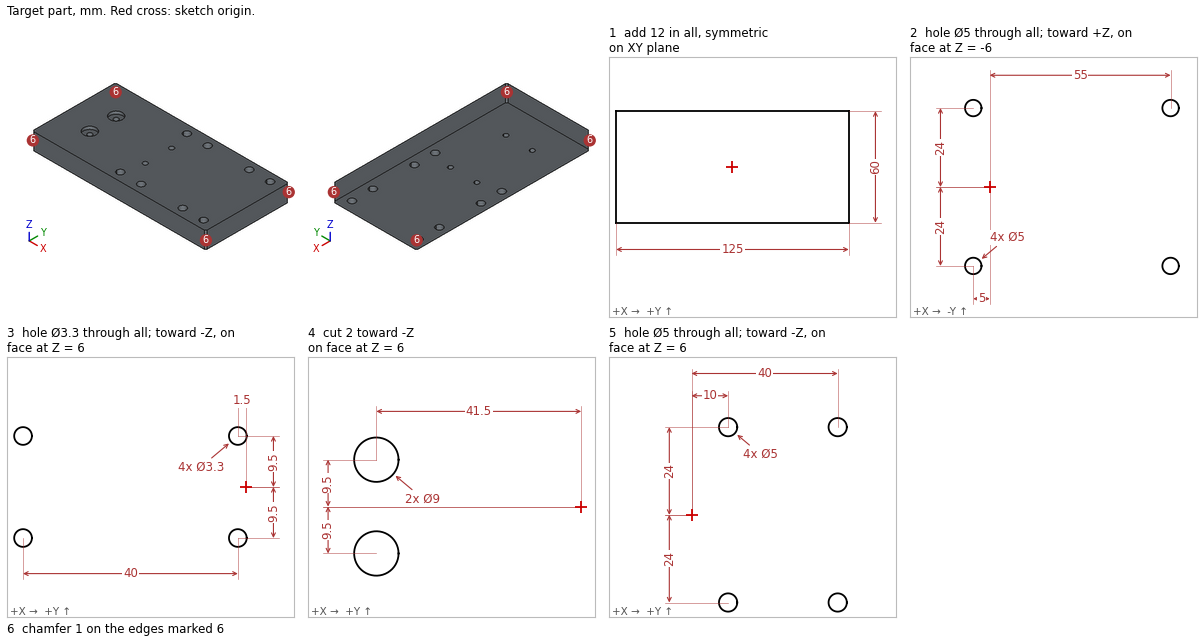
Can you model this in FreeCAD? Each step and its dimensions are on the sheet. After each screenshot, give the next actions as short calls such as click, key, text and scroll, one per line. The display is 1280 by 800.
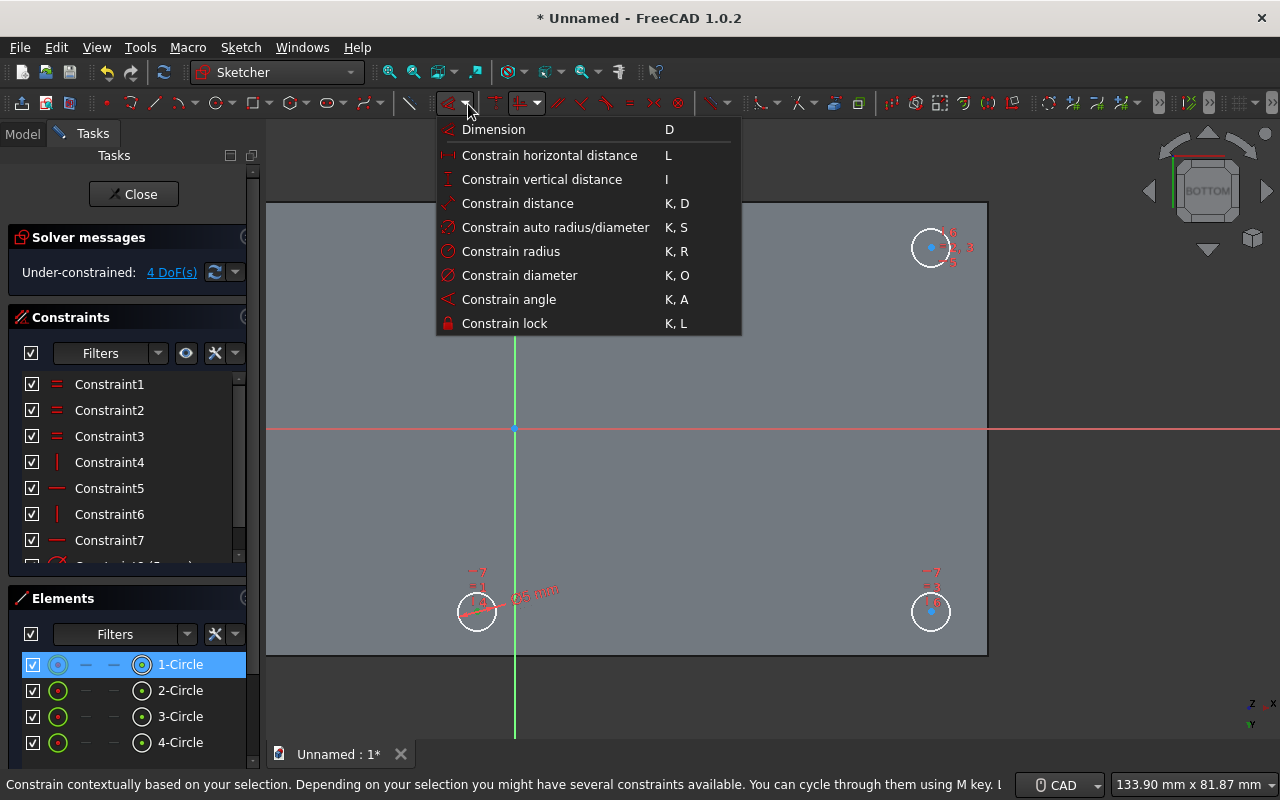
click(589, 155)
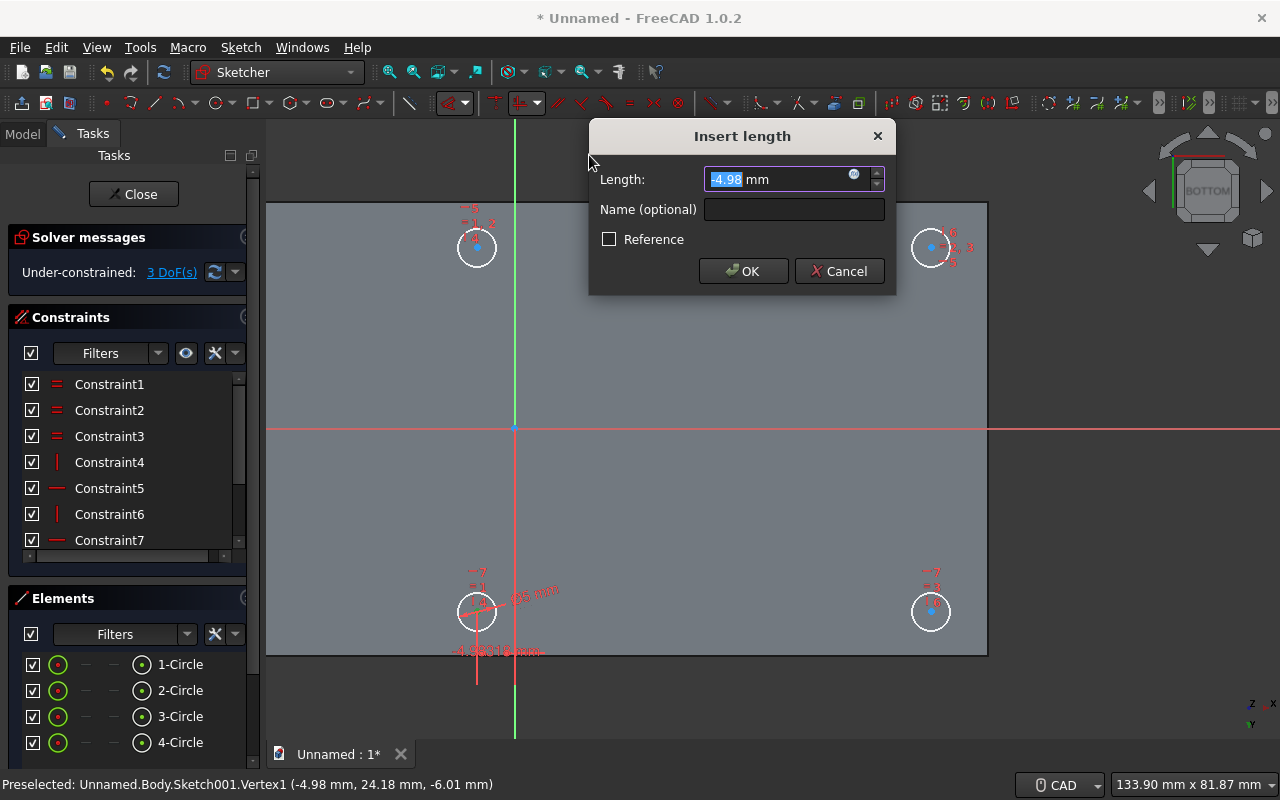
text(-5)
key(Return)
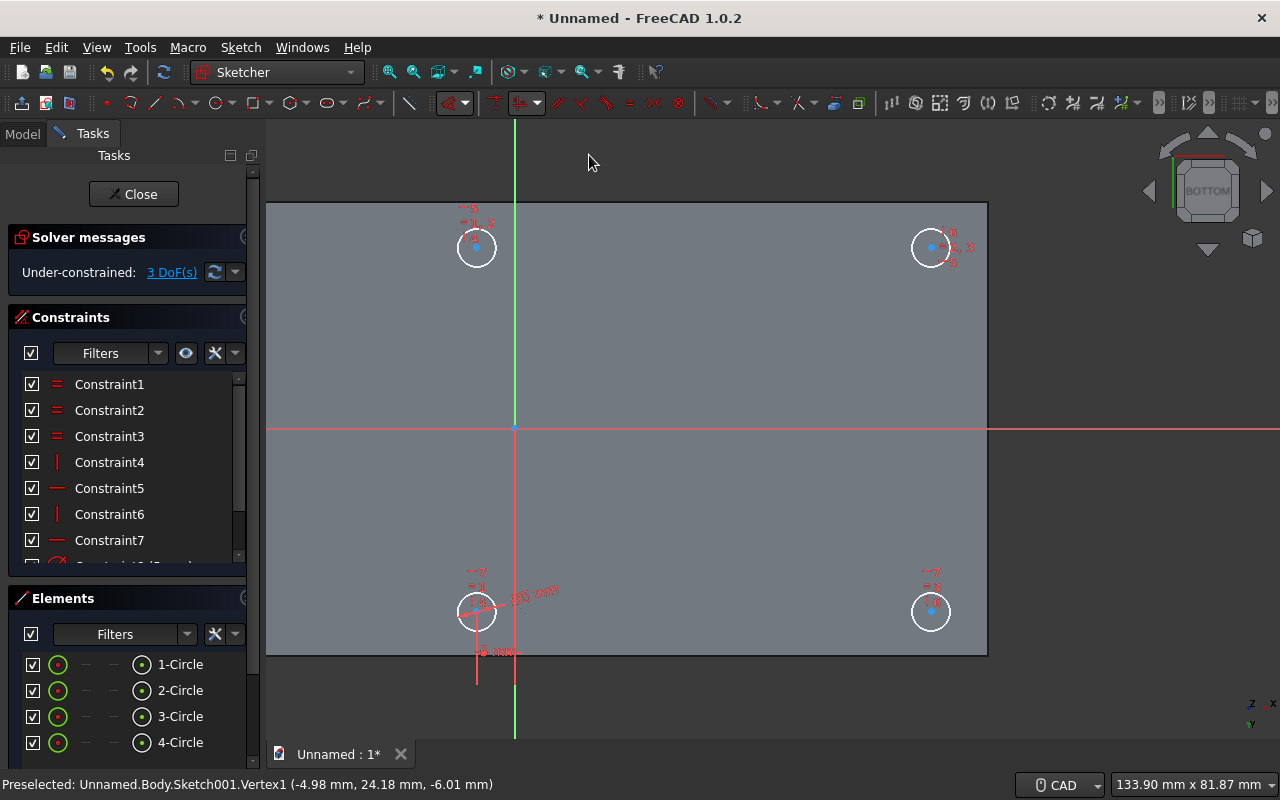
click(477, 612)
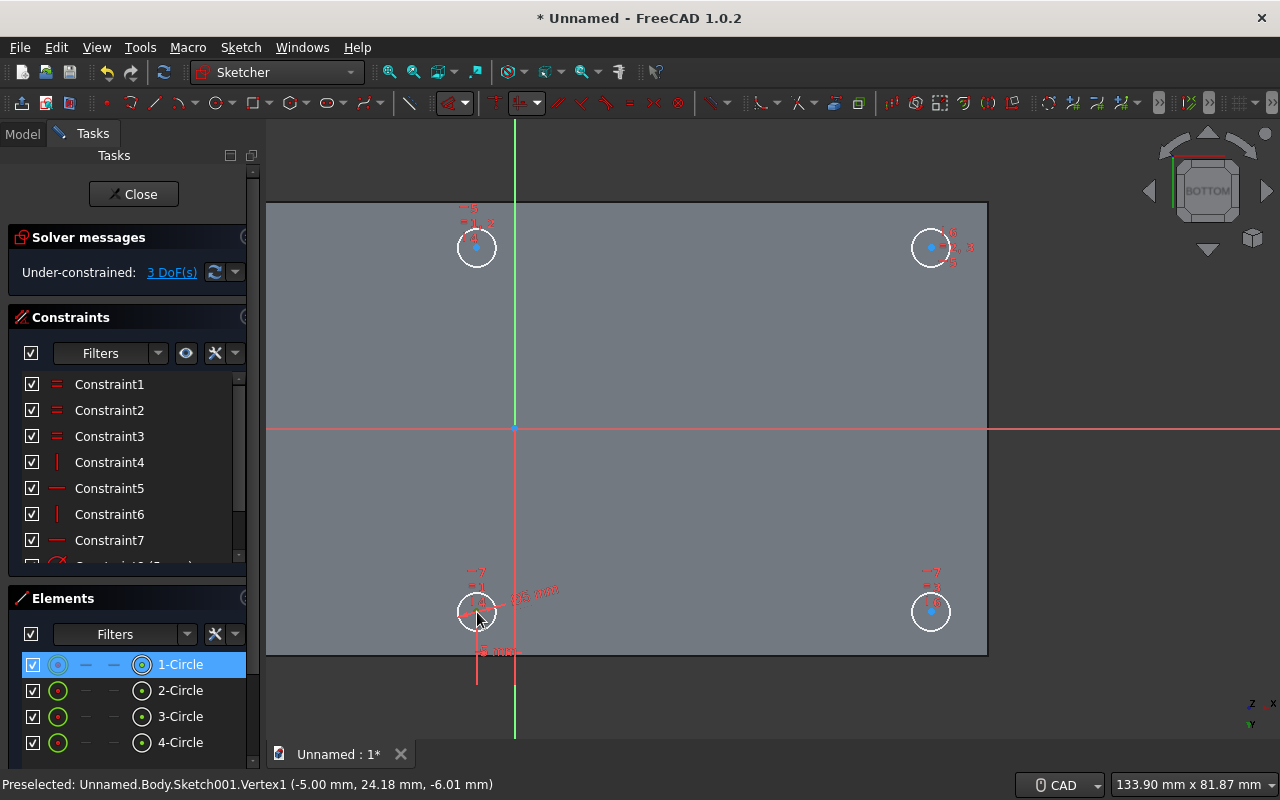
key(i)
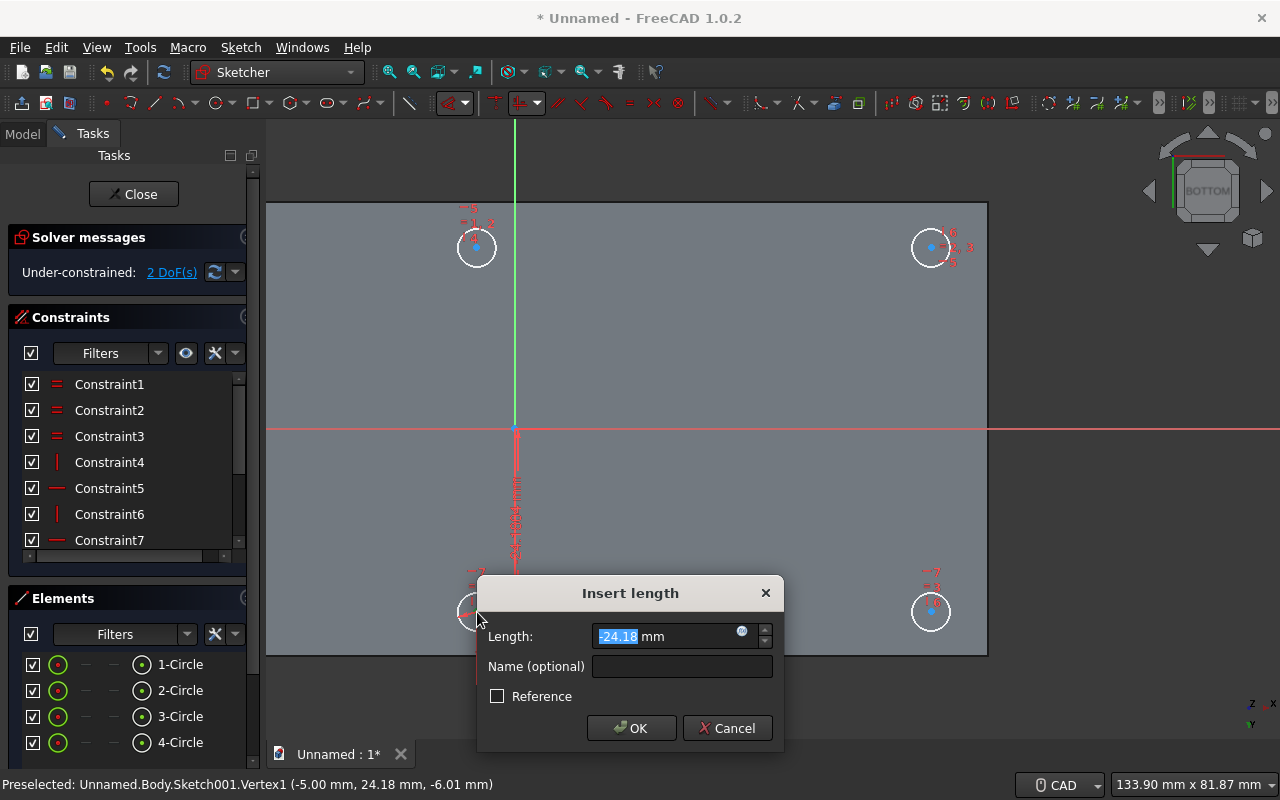
text(-24)
key(Return)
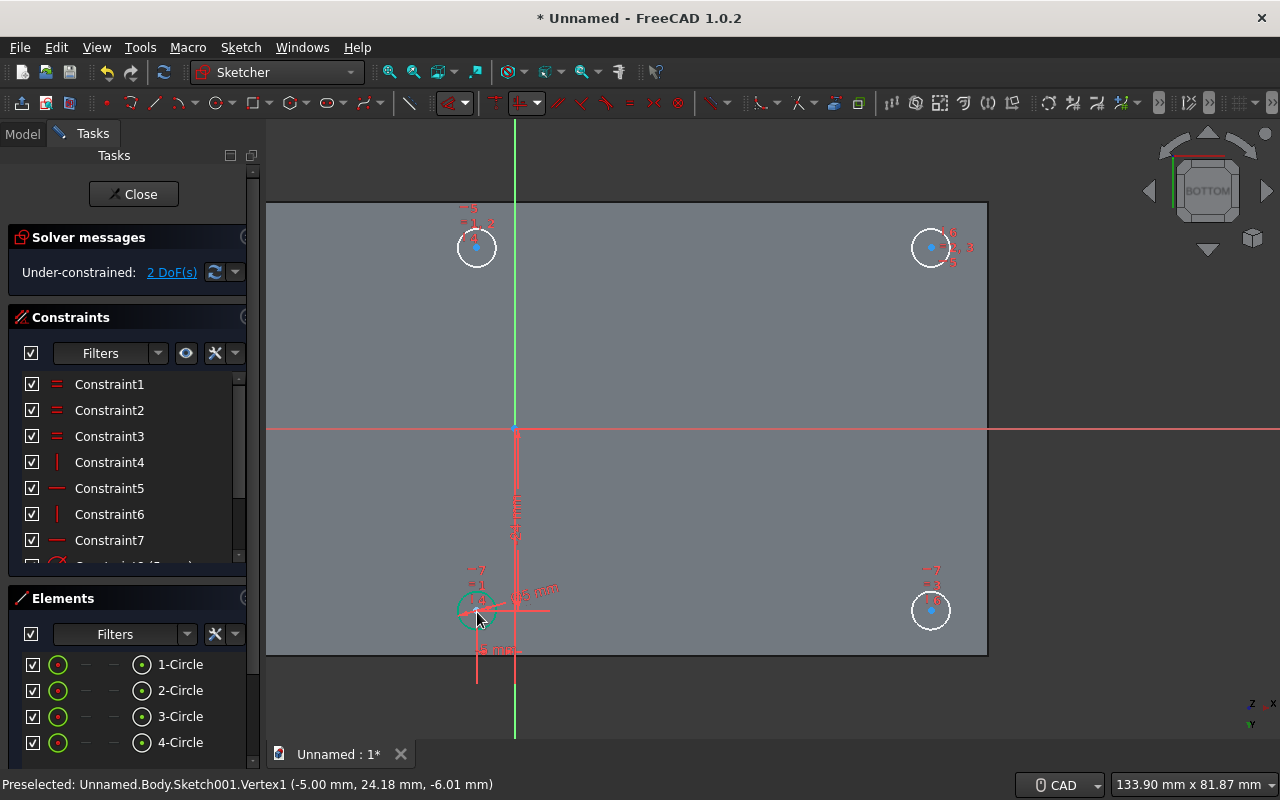
click(477, 248)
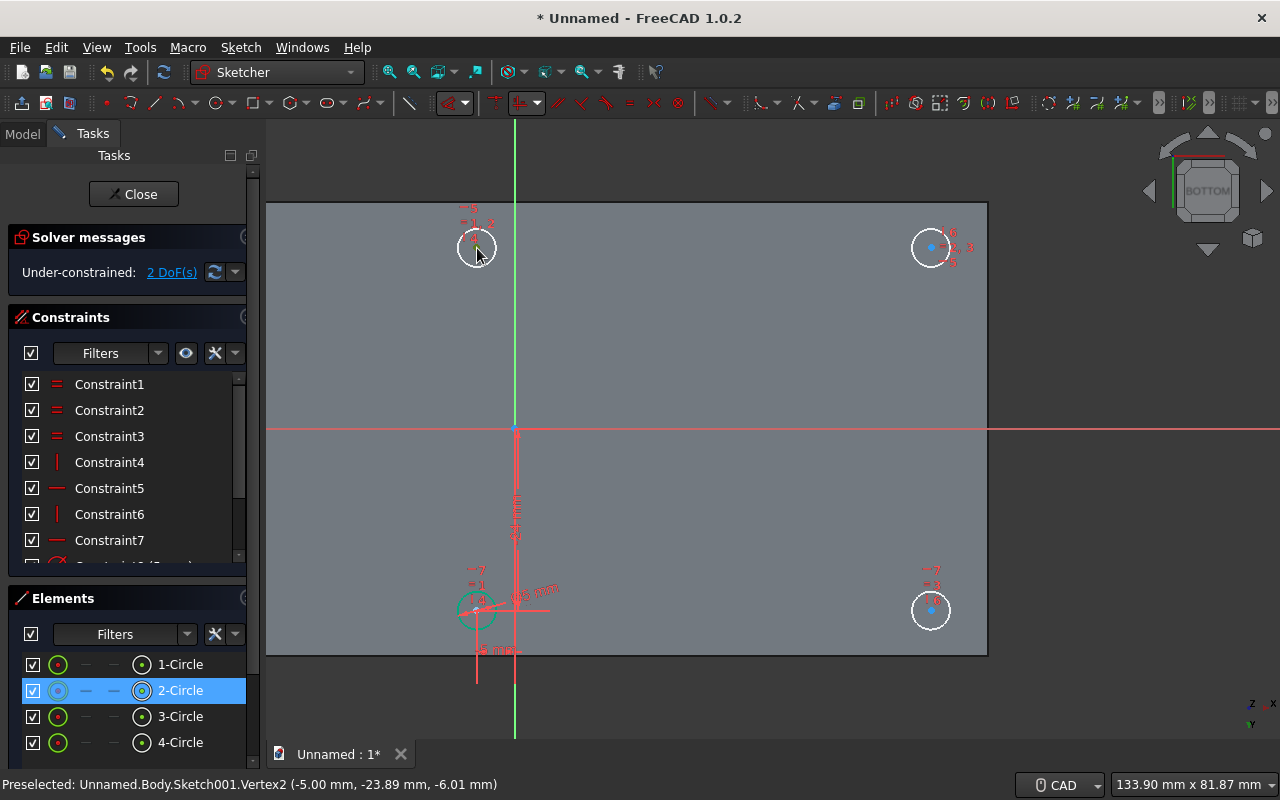
key(i)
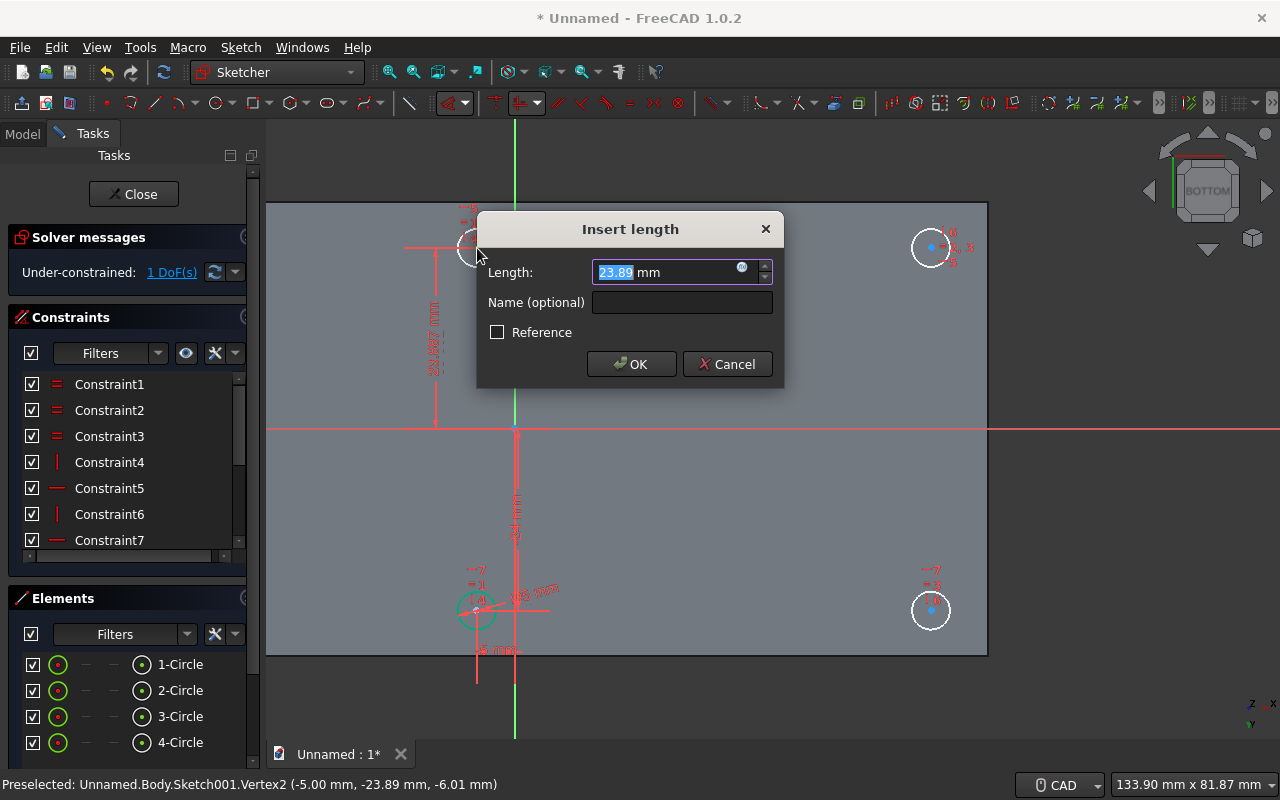
text(24)
key(Return)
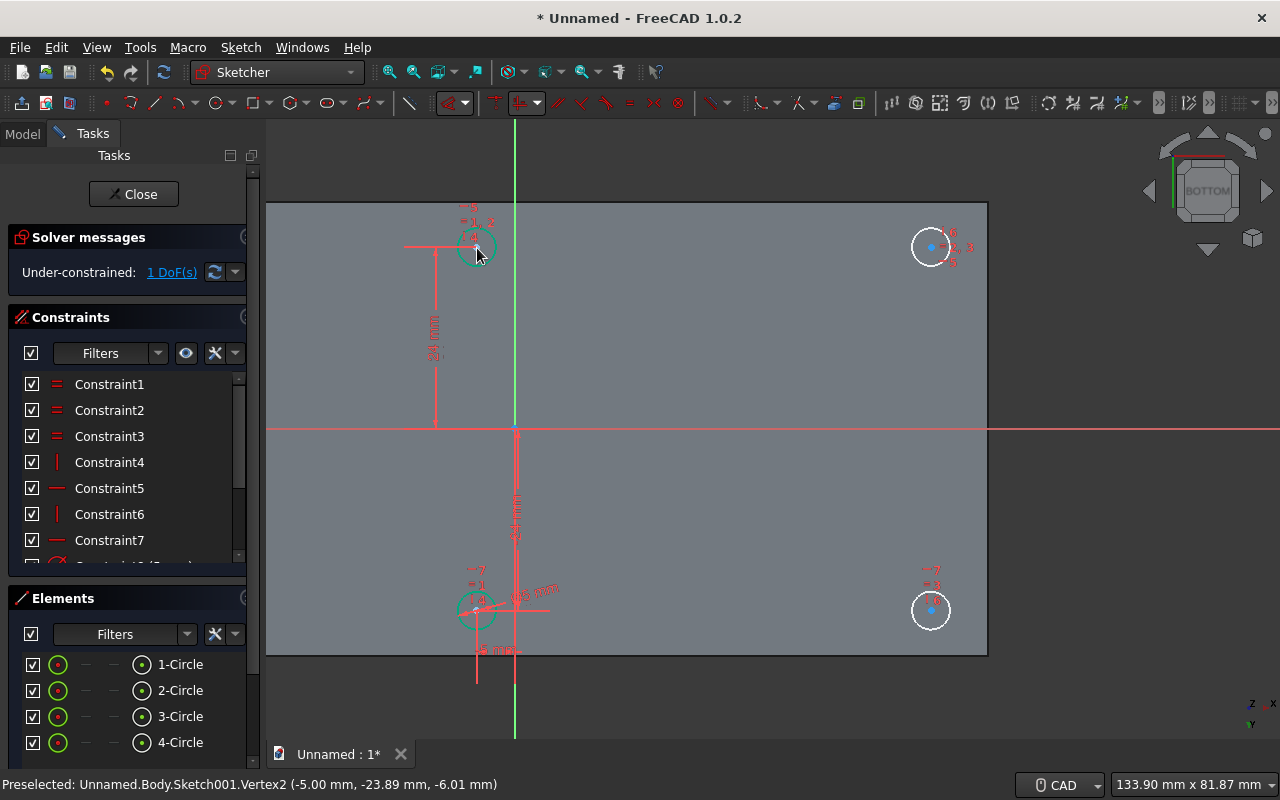
click(931, 247)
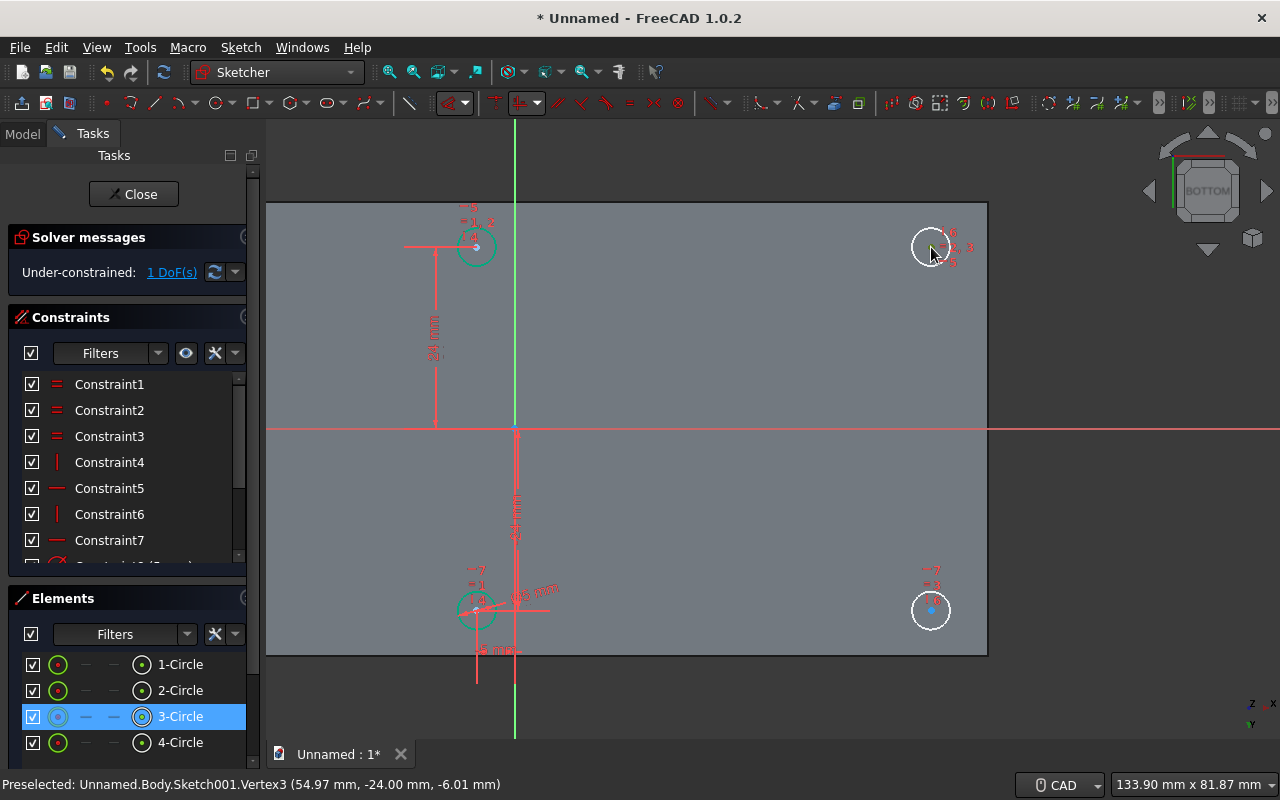
key(l)